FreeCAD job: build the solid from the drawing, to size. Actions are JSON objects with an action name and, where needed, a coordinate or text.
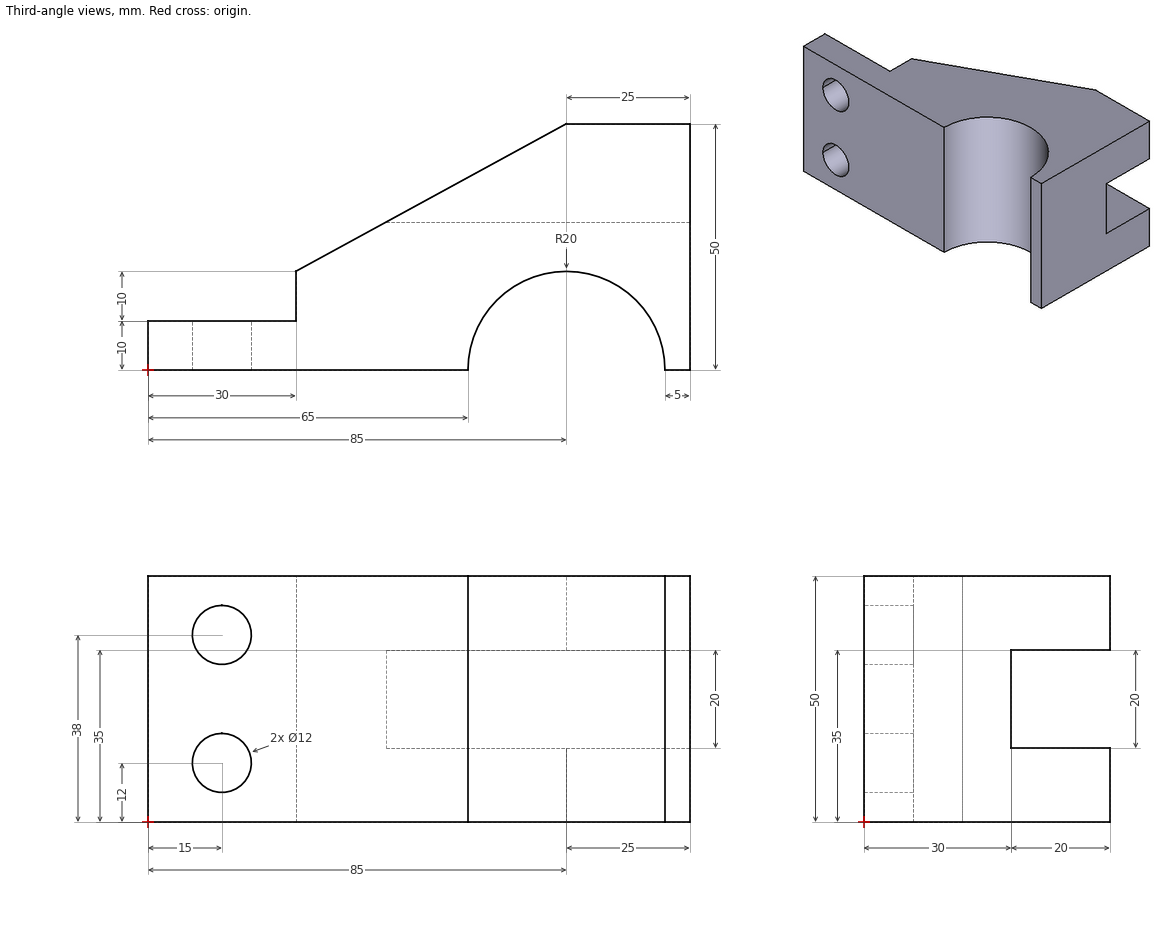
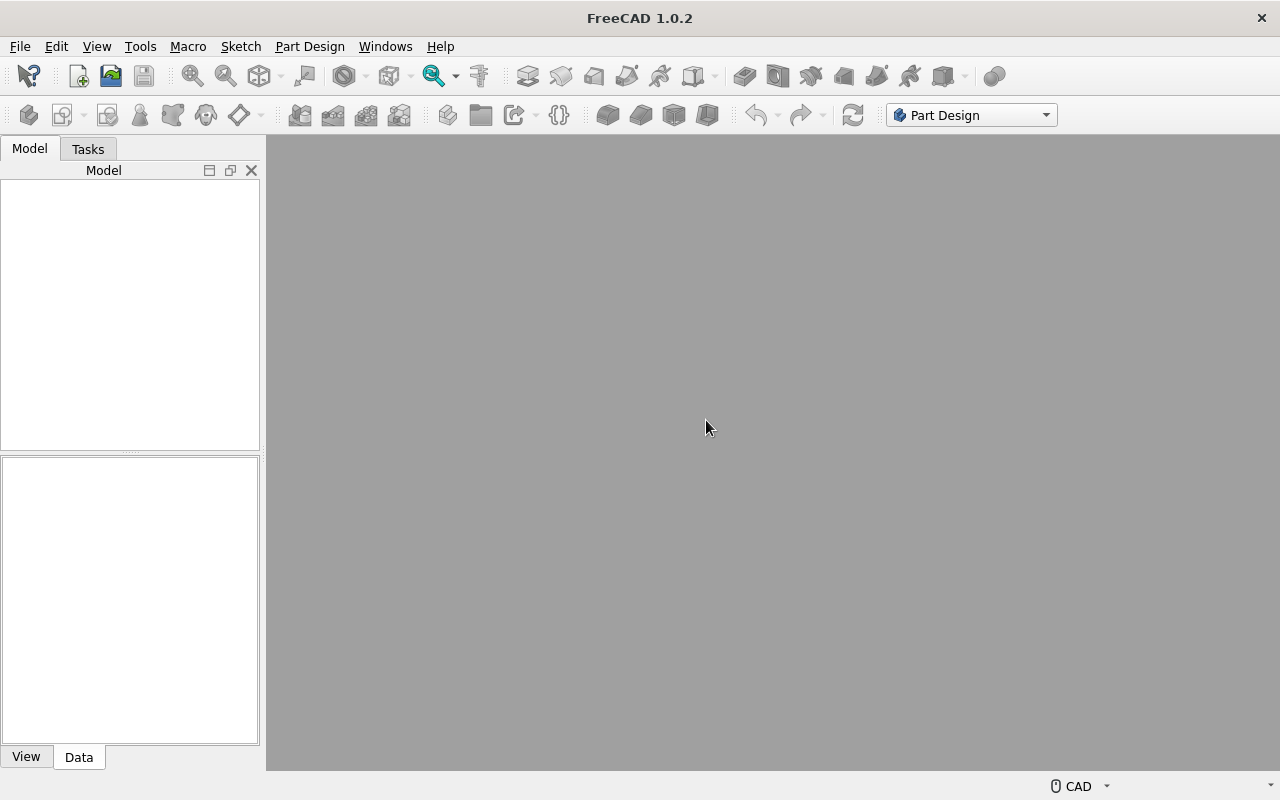
{"action": "left_click", "coordinate": [78, 76]}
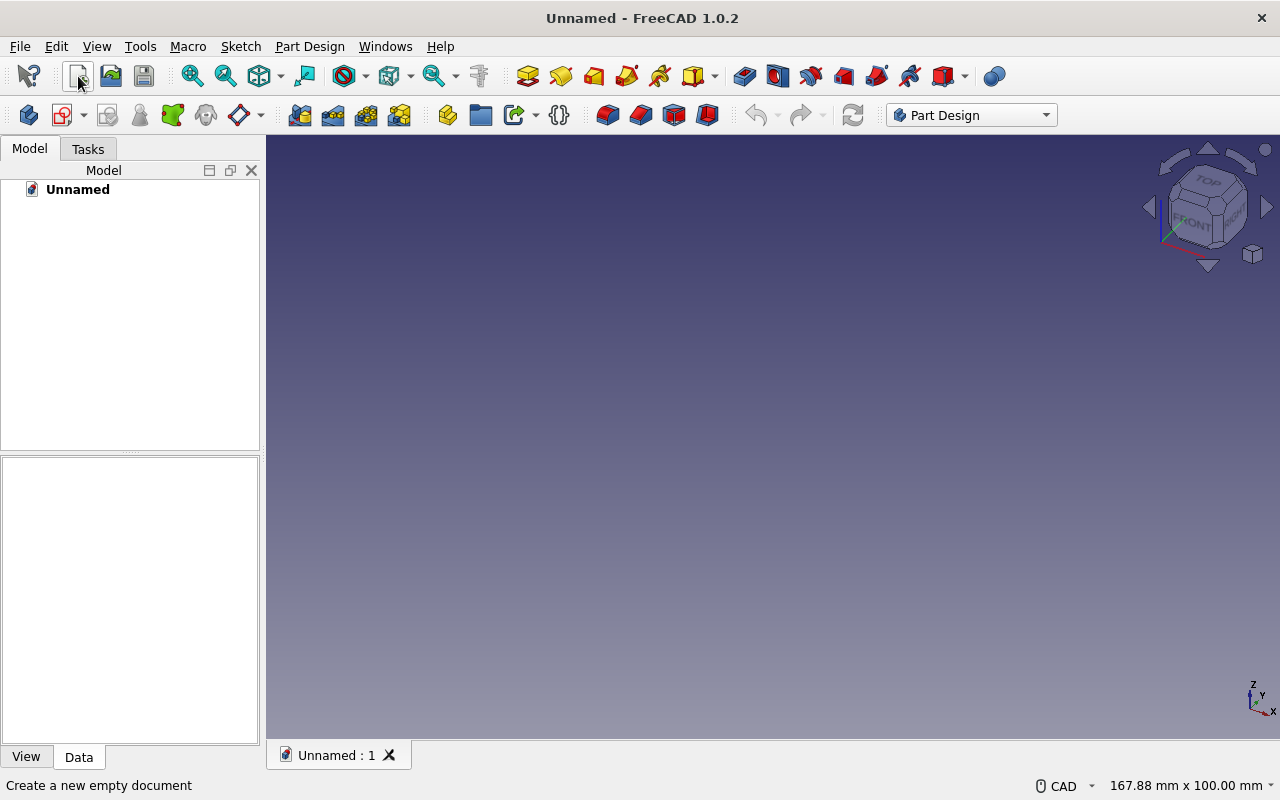
{"action": "left_click", "coordinate": [62, 116]}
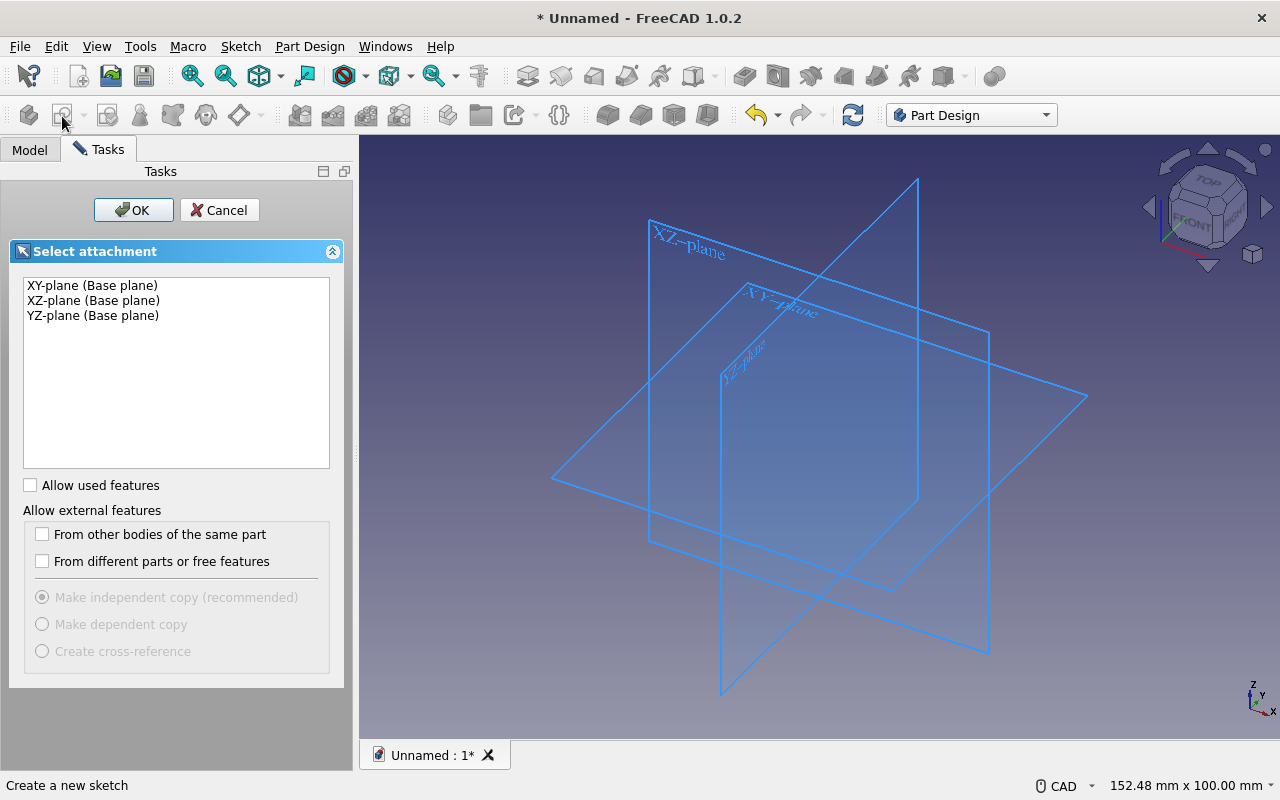
{"action": "left_click", "coordinate": [84, 286]}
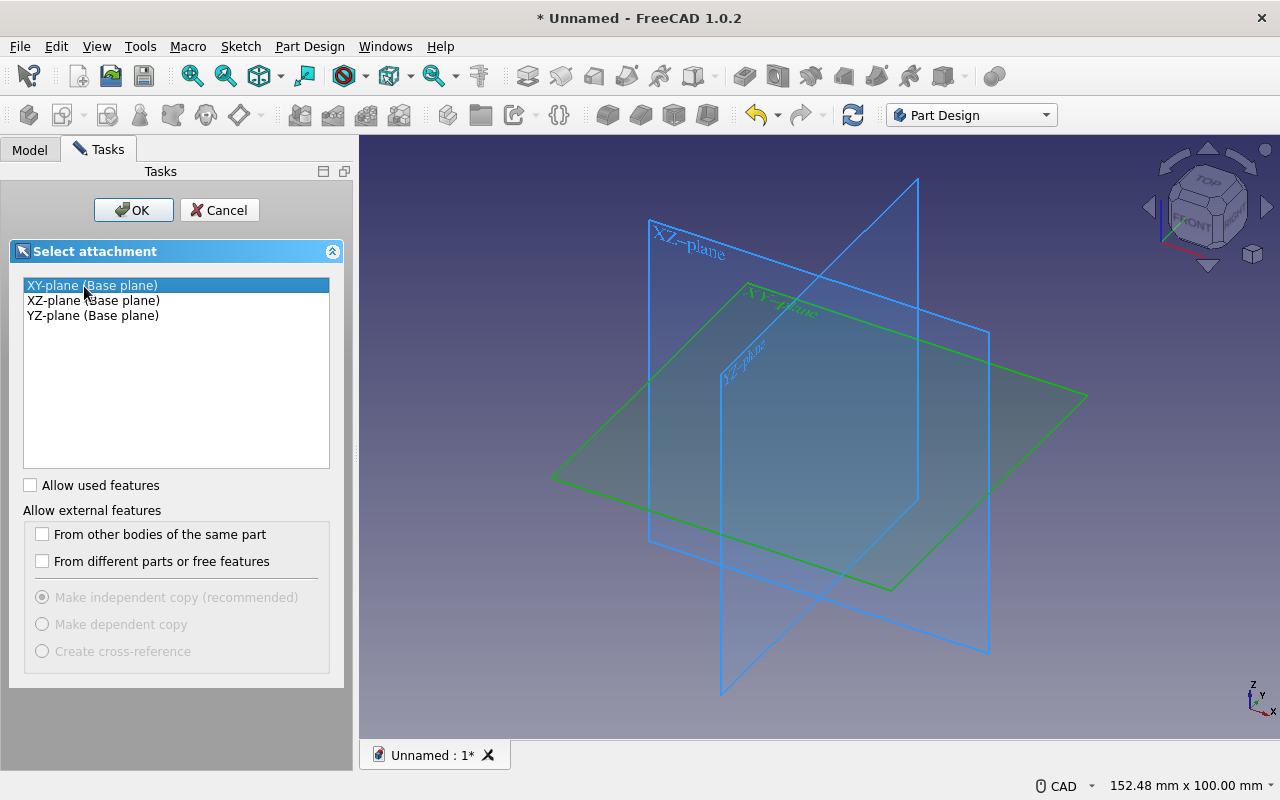
{"action": "left_click", "coordinate": [134, 210]}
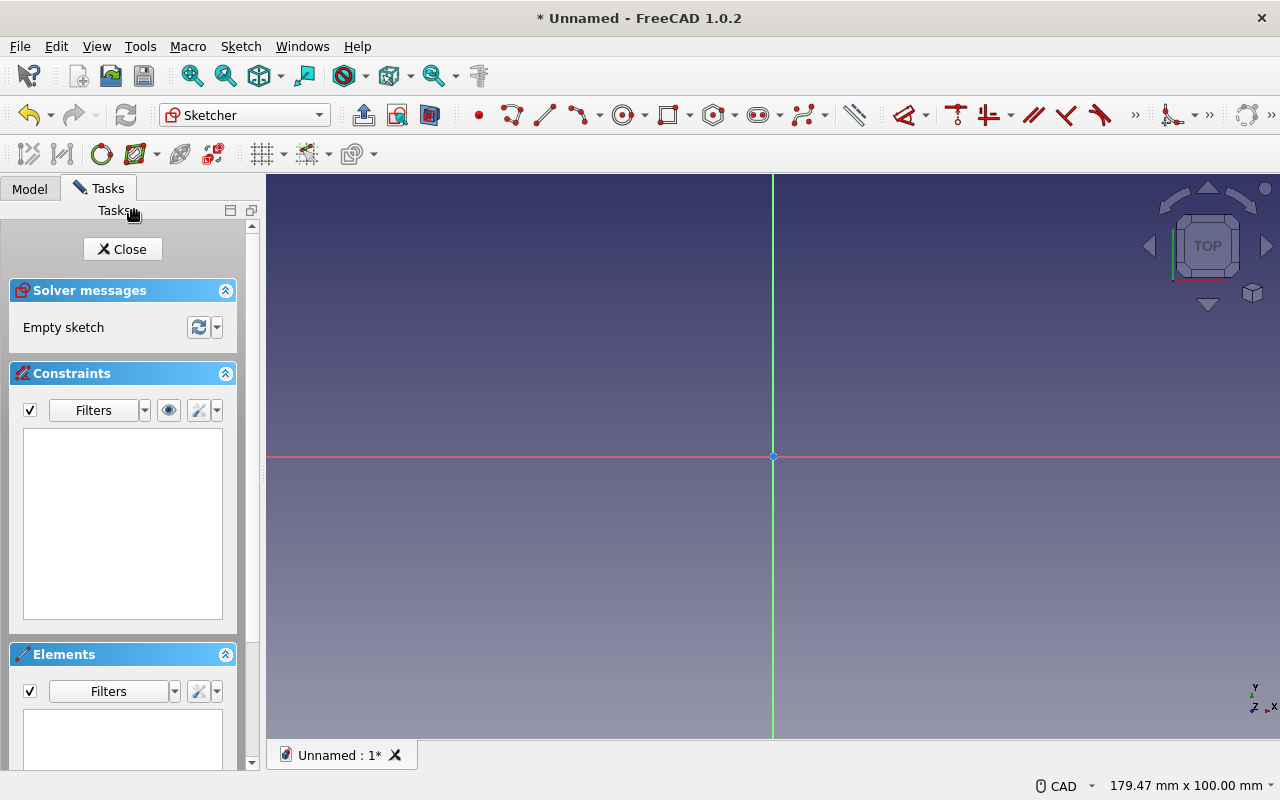
{"action": "scroll", "coordinate": [294, 711], "scroll_direction": "down", "scroll_amount": 2}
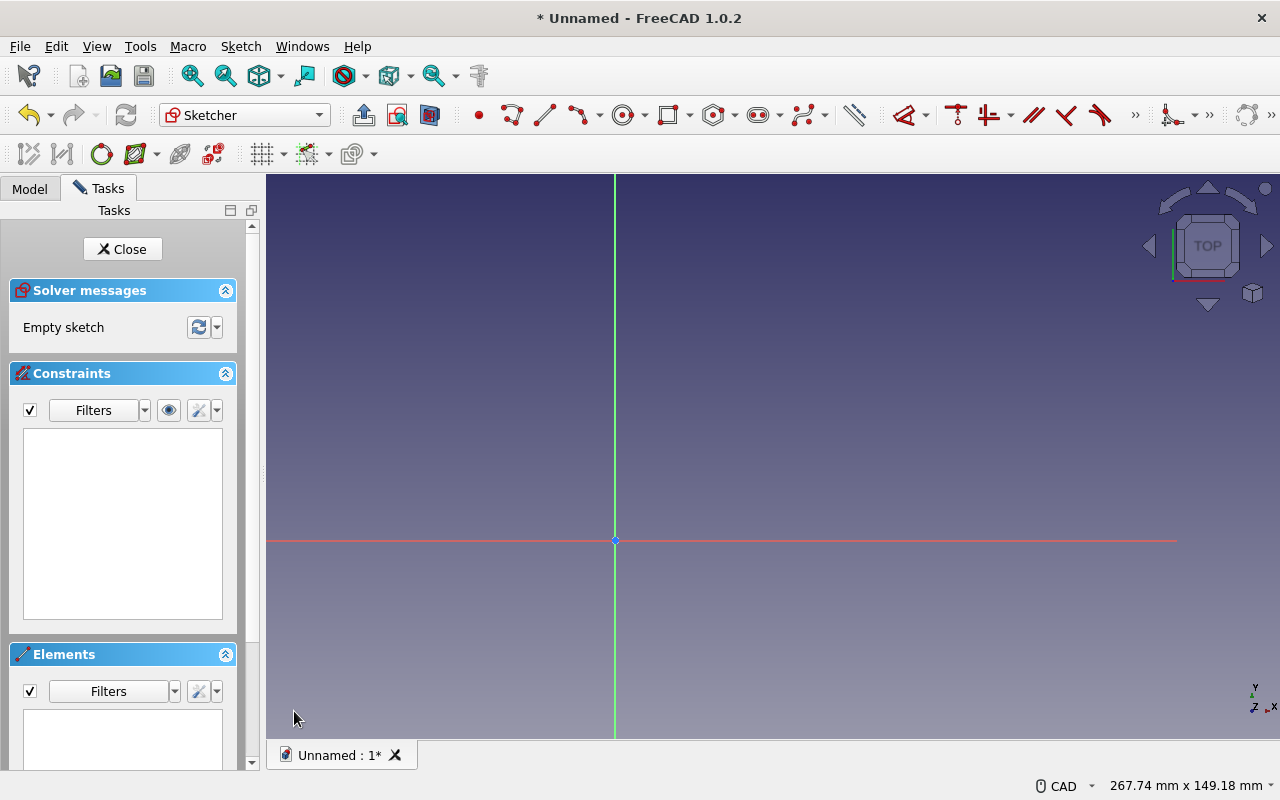
{"action": "scroll", "coordinate": [1065, 425], "scroll_direction": "up", "scroll_amount": 2}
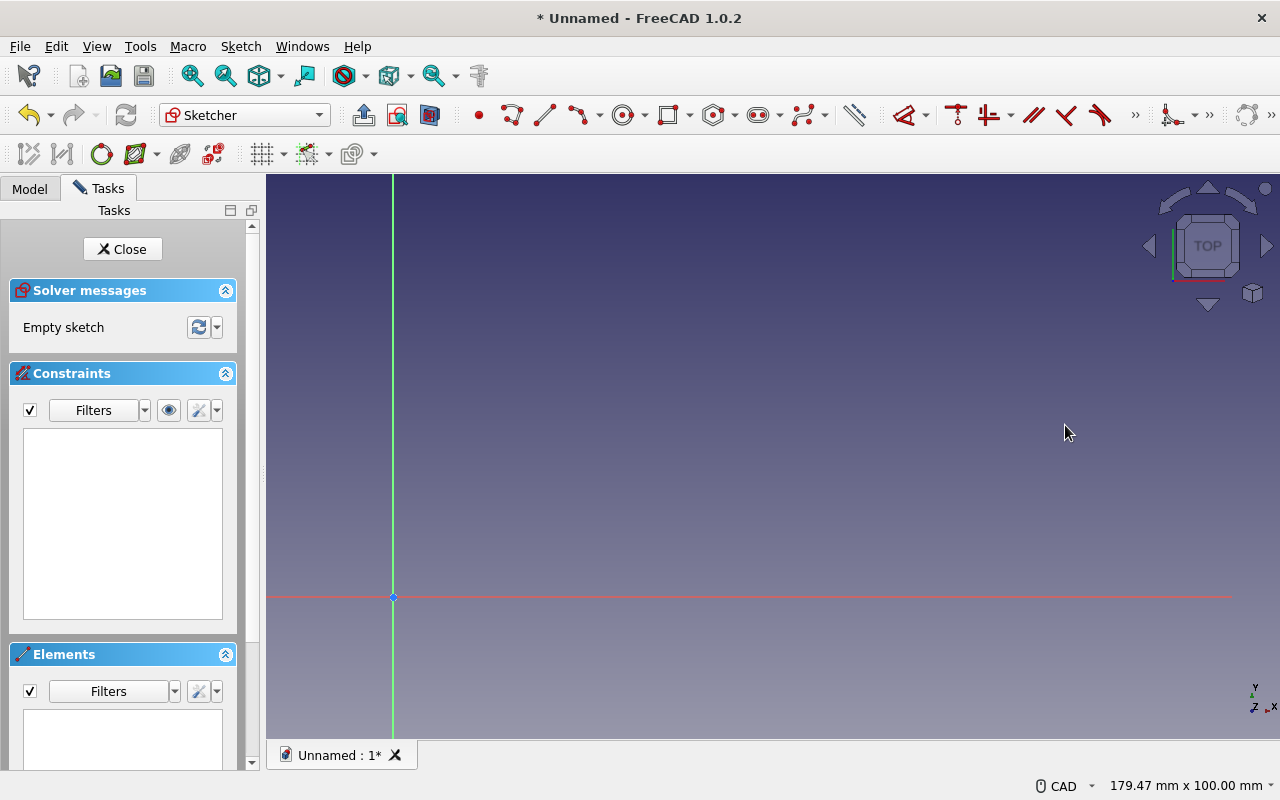
{"action": "left_click", "coordinate": [512, 116]}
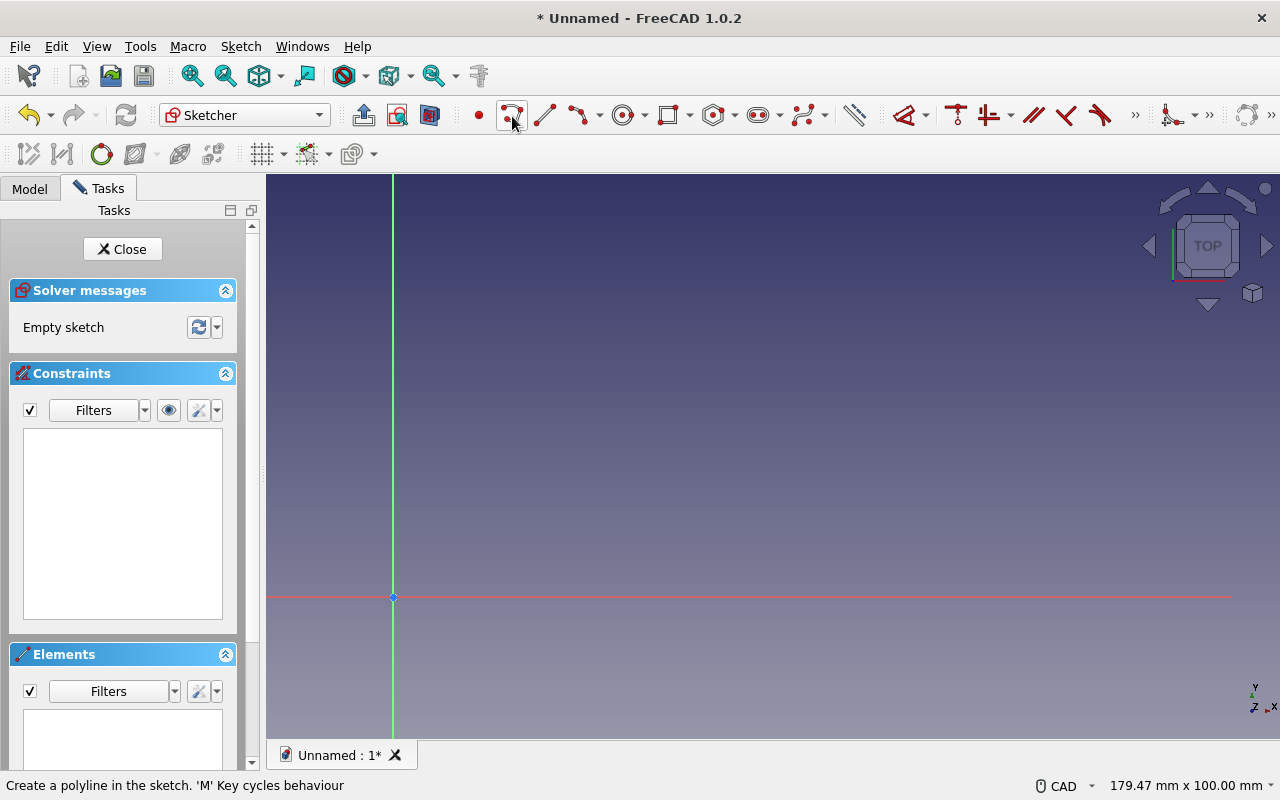
{"action": "left_click", "coordinate": [987, 597]}
{"action": "left_click", "coordinate": [1015, 588]}
{"action": "left_click", "coordinate": [1015, 315]}
{"action": "left_click", "coordinate": [874, 315]}
{"action": "left_click", "coordinate": [563, 484]}
{"action": "left_click", "coordinate": [563, 541]}
{"action": "left_click", "coordinate": [393, 541]}
{"action": "left_click", "coordinate": [393, 597]}
{"action": "left_click", "coordinate": [761, 588]}
{"action": "right_click", "coordinate": [761, 588]}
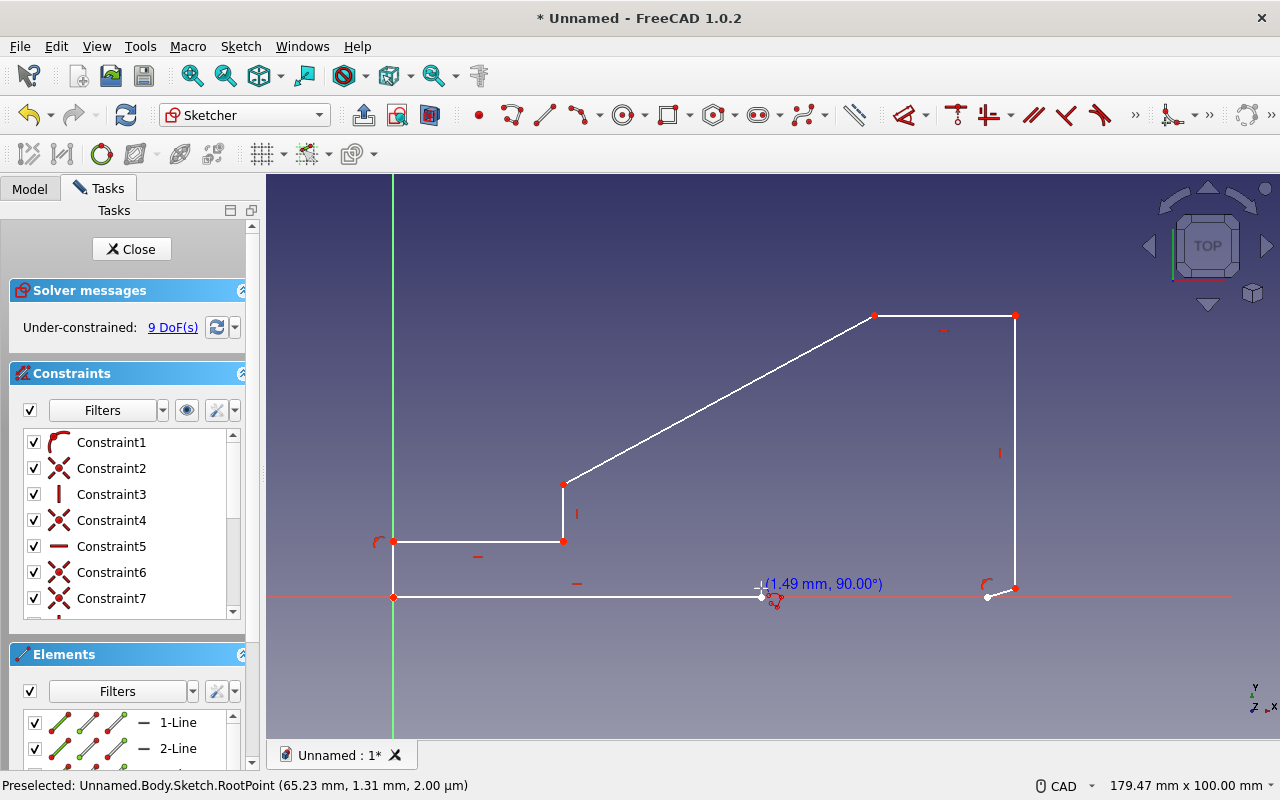
{"action": "left_click", "coordinate": [578, 116]}